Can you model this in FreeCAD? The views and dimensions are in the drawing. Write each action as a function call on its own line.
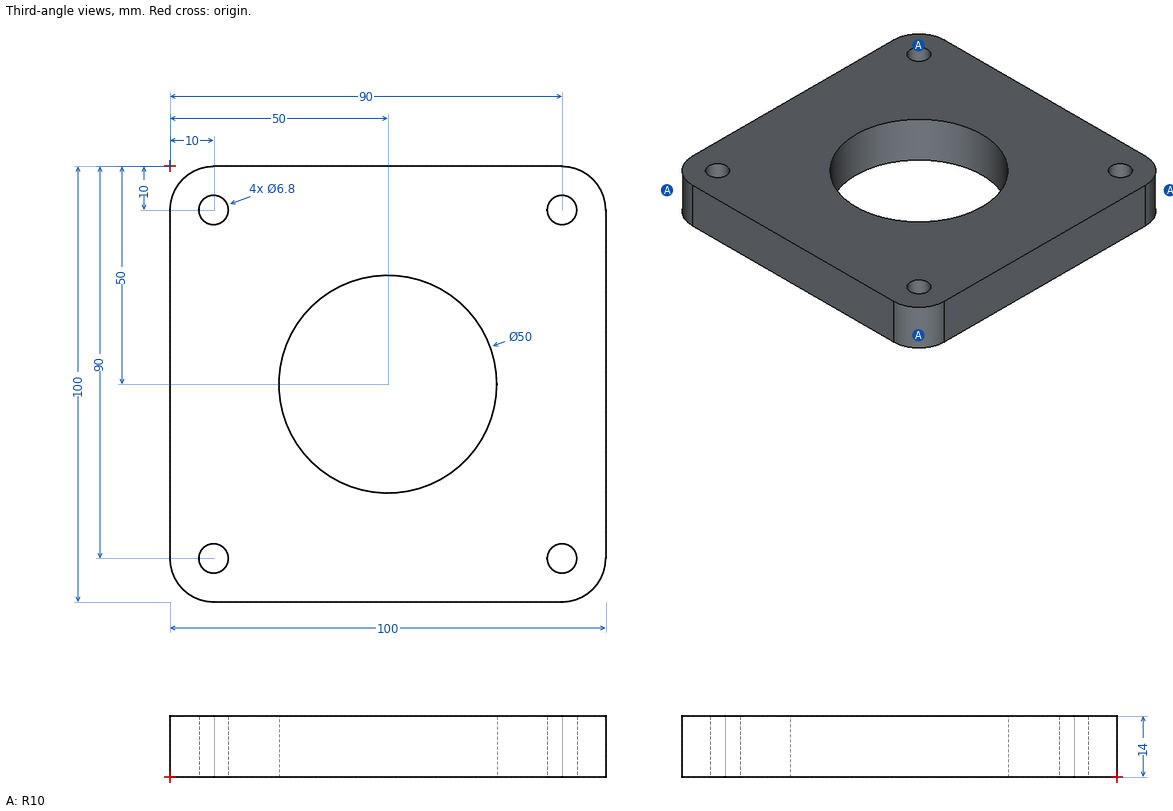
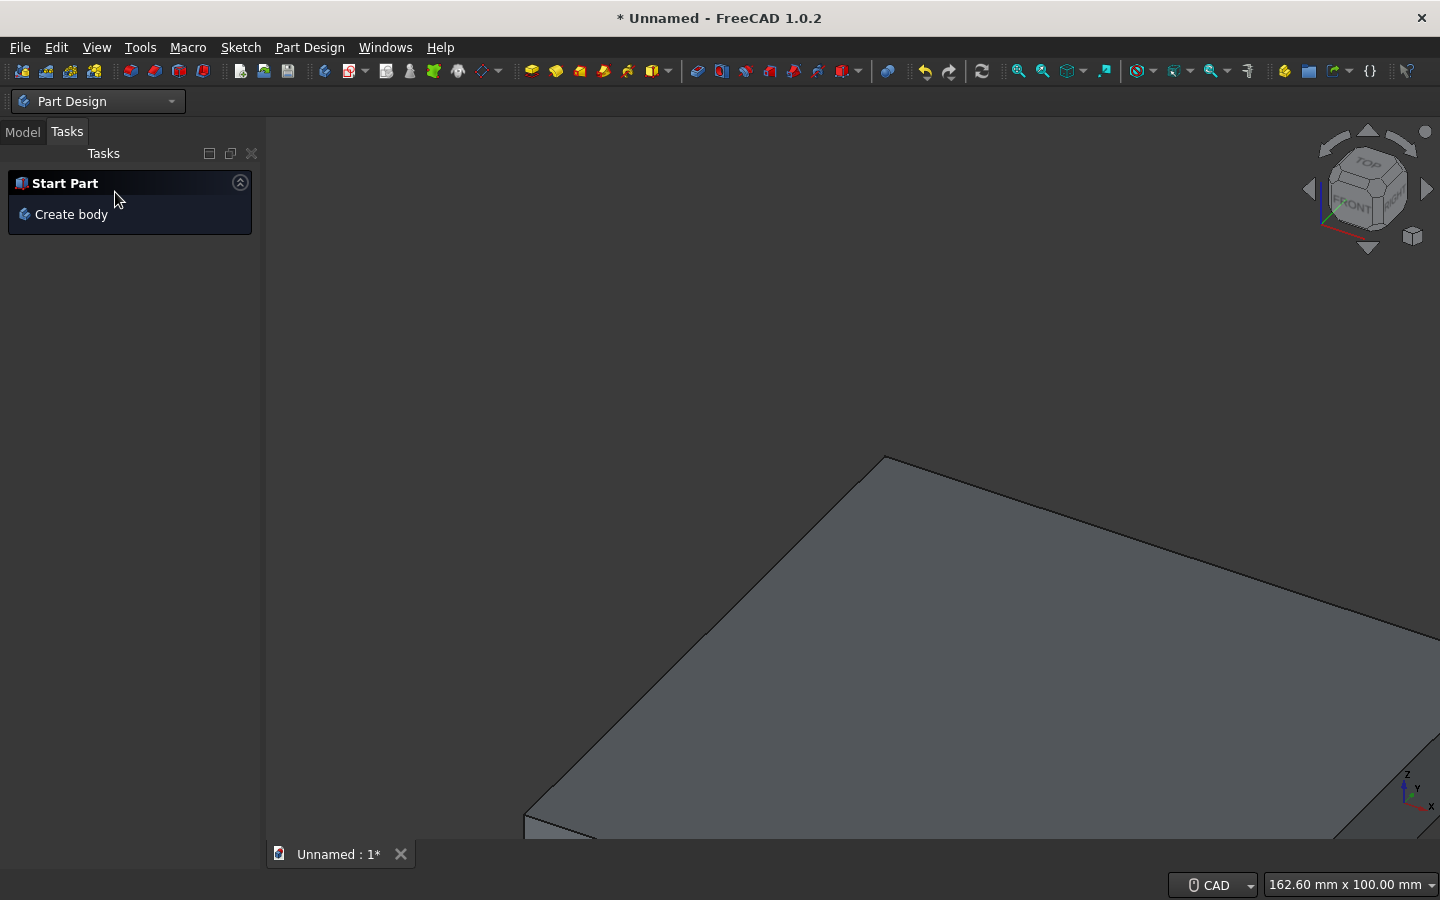
click(1020, 72)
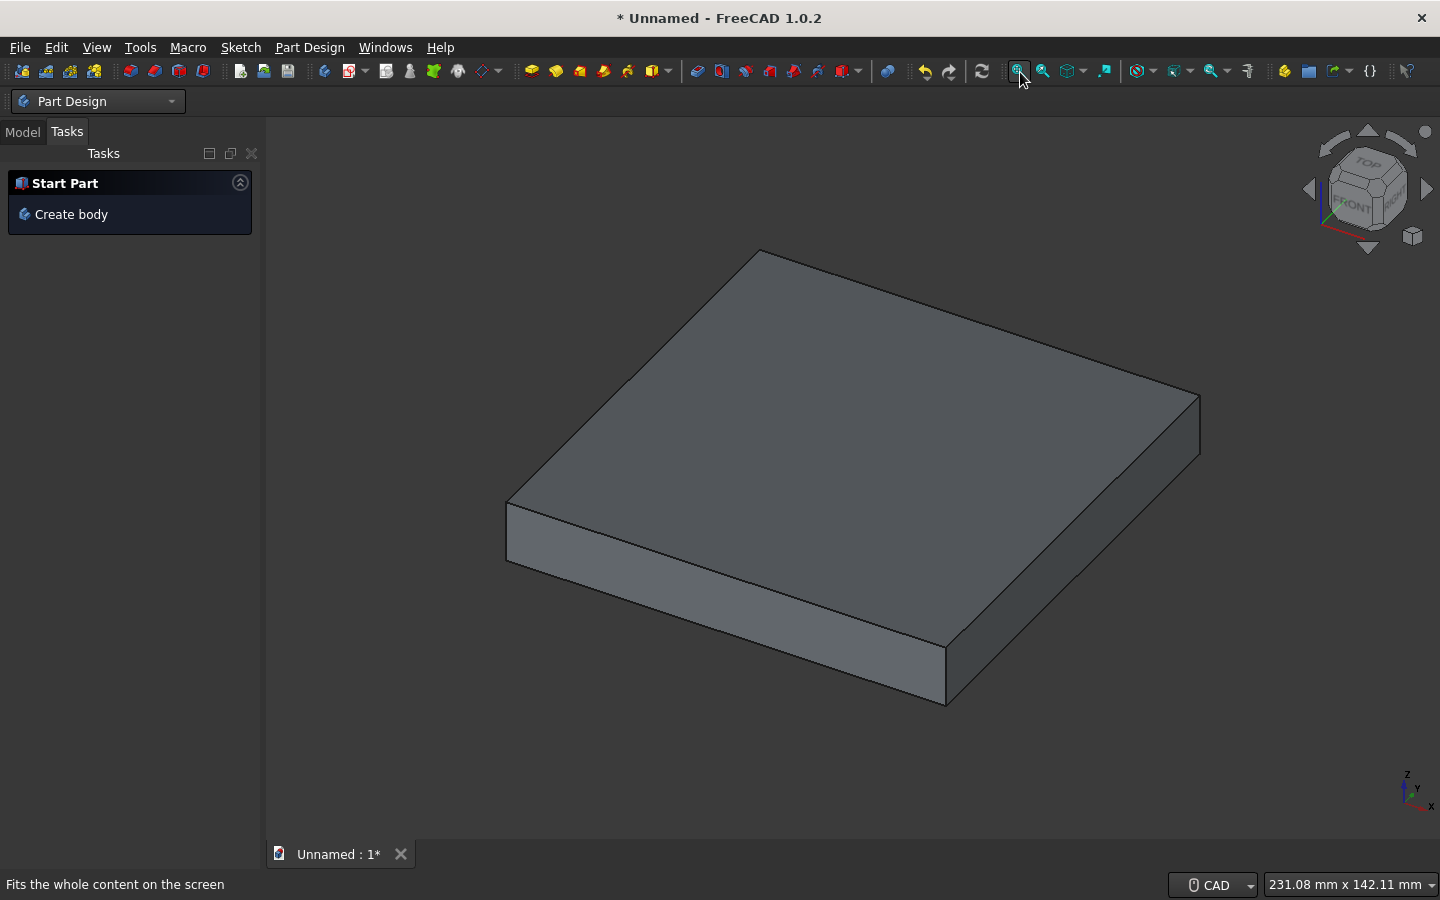
click(853, 448)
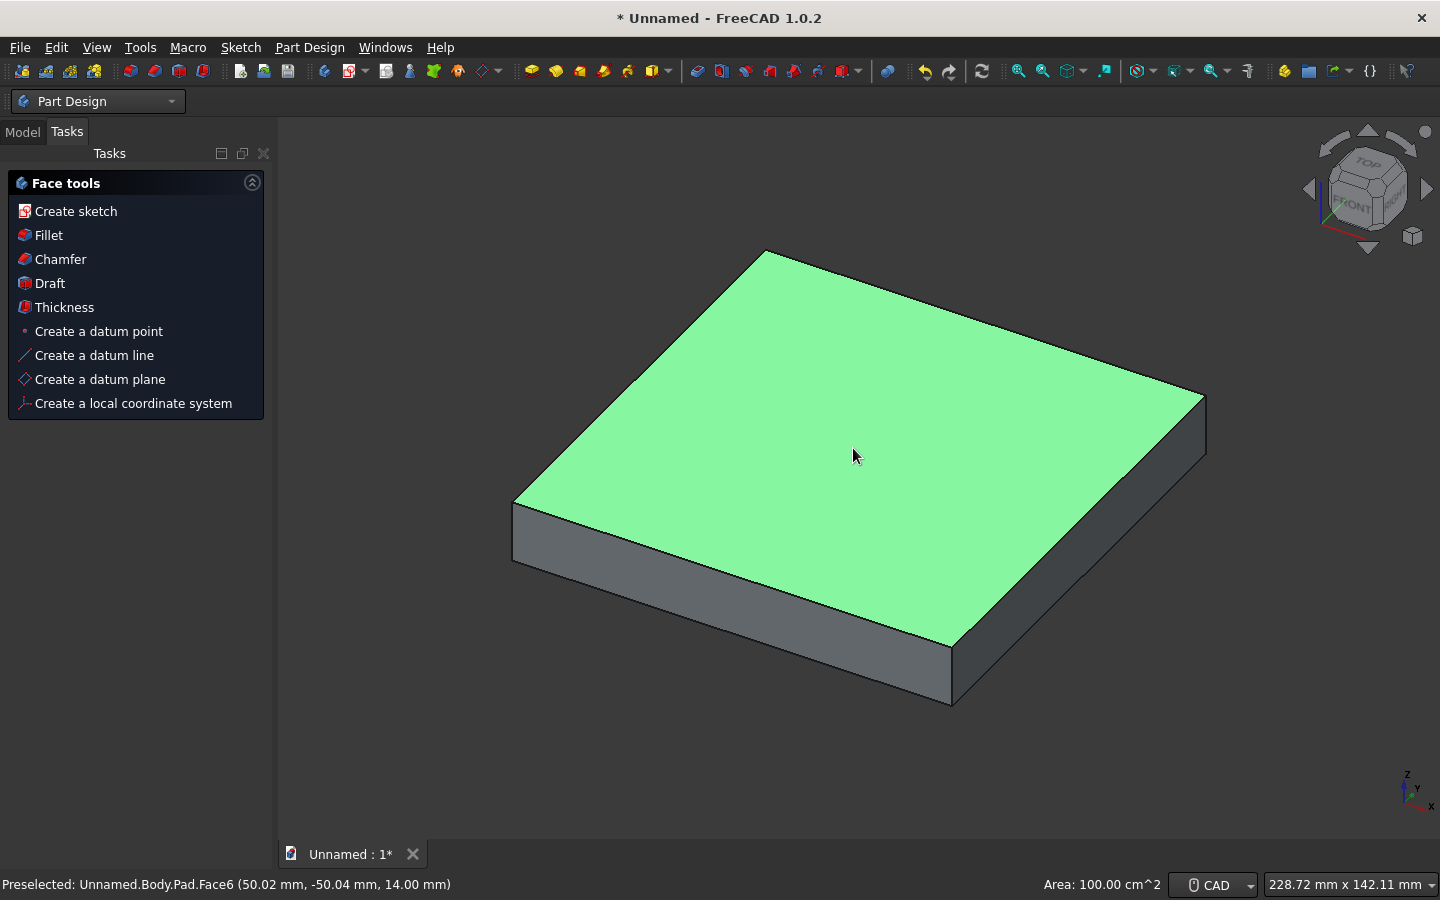
click(350, 72)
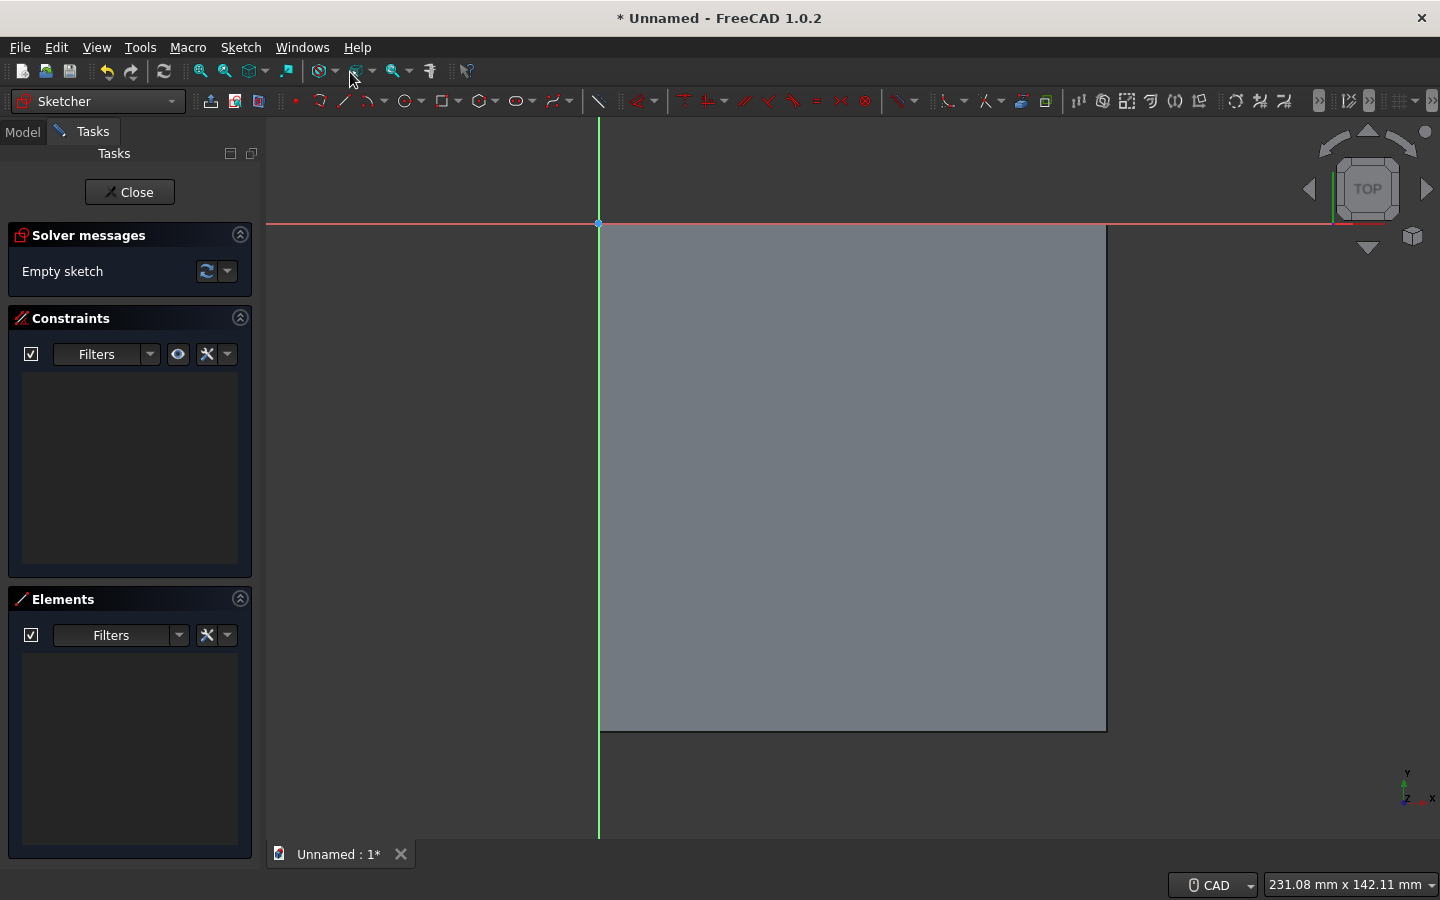
click(406, 102)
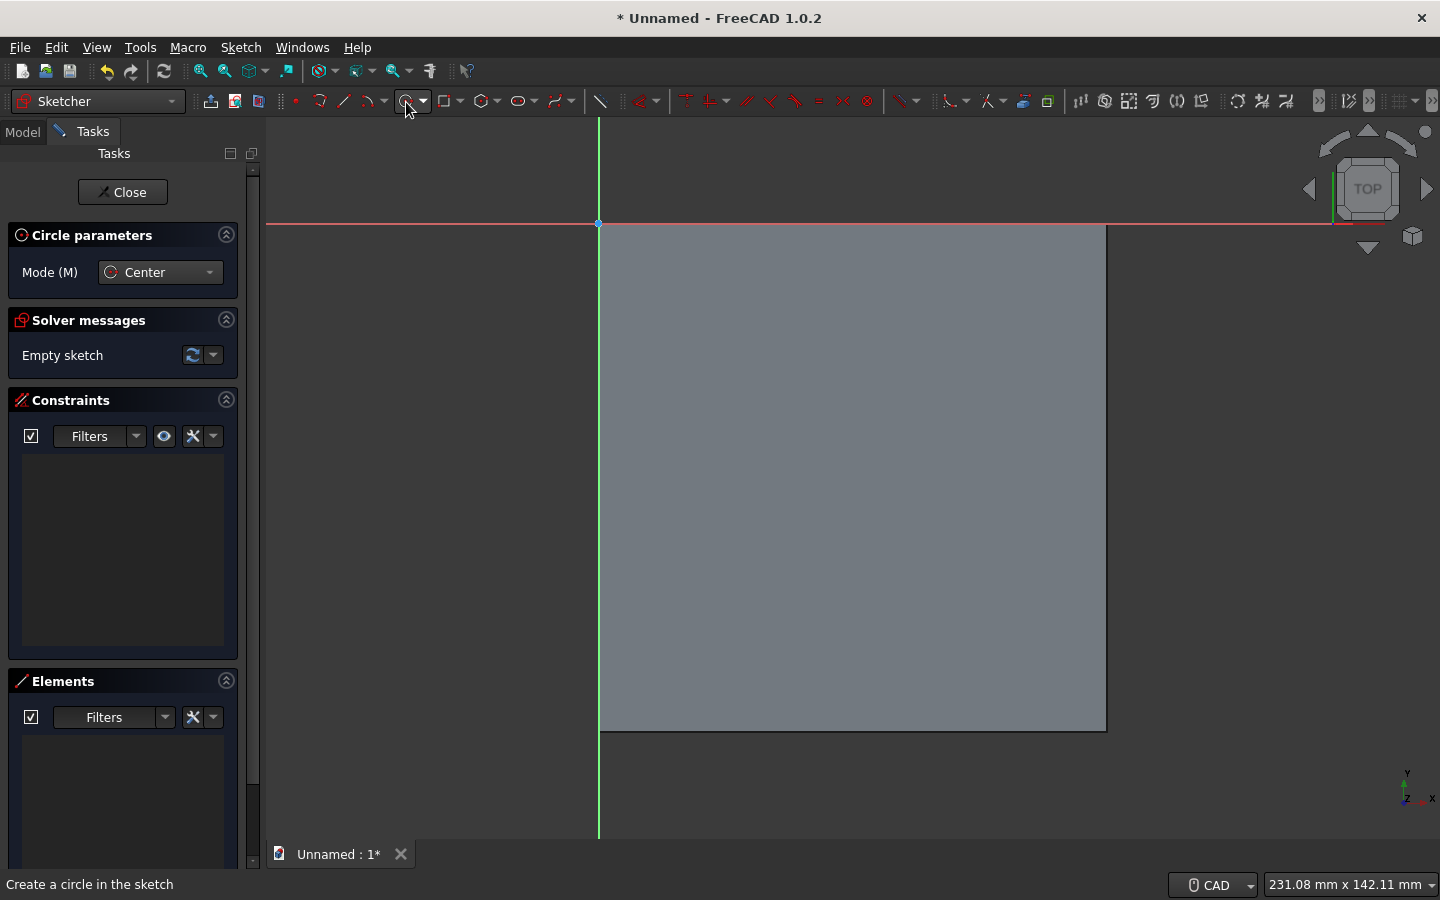
click(853, 478)
click(943, 388)
key(Escape)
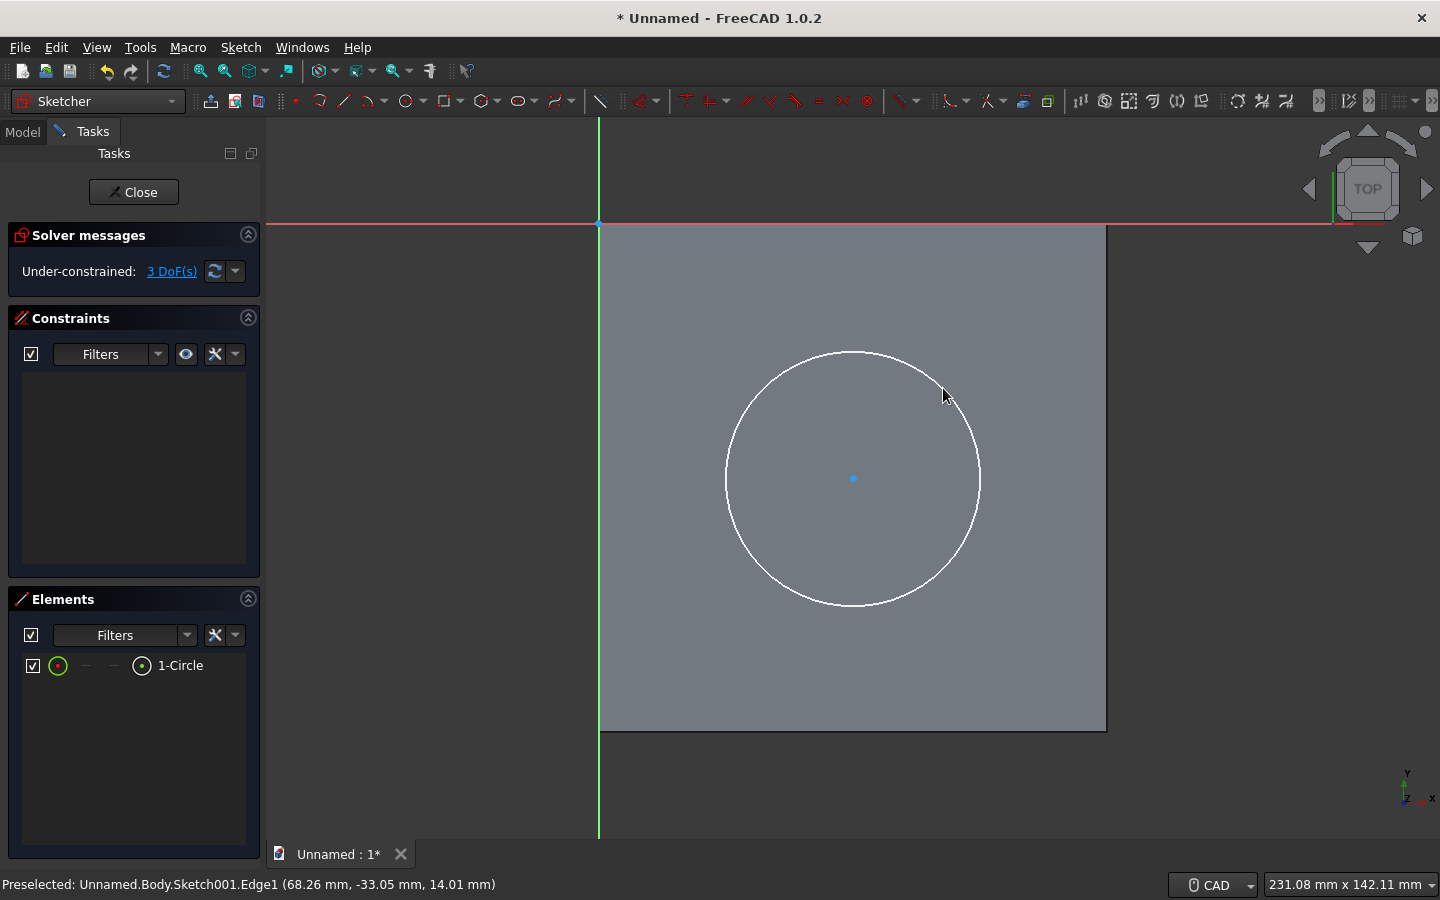
key(d)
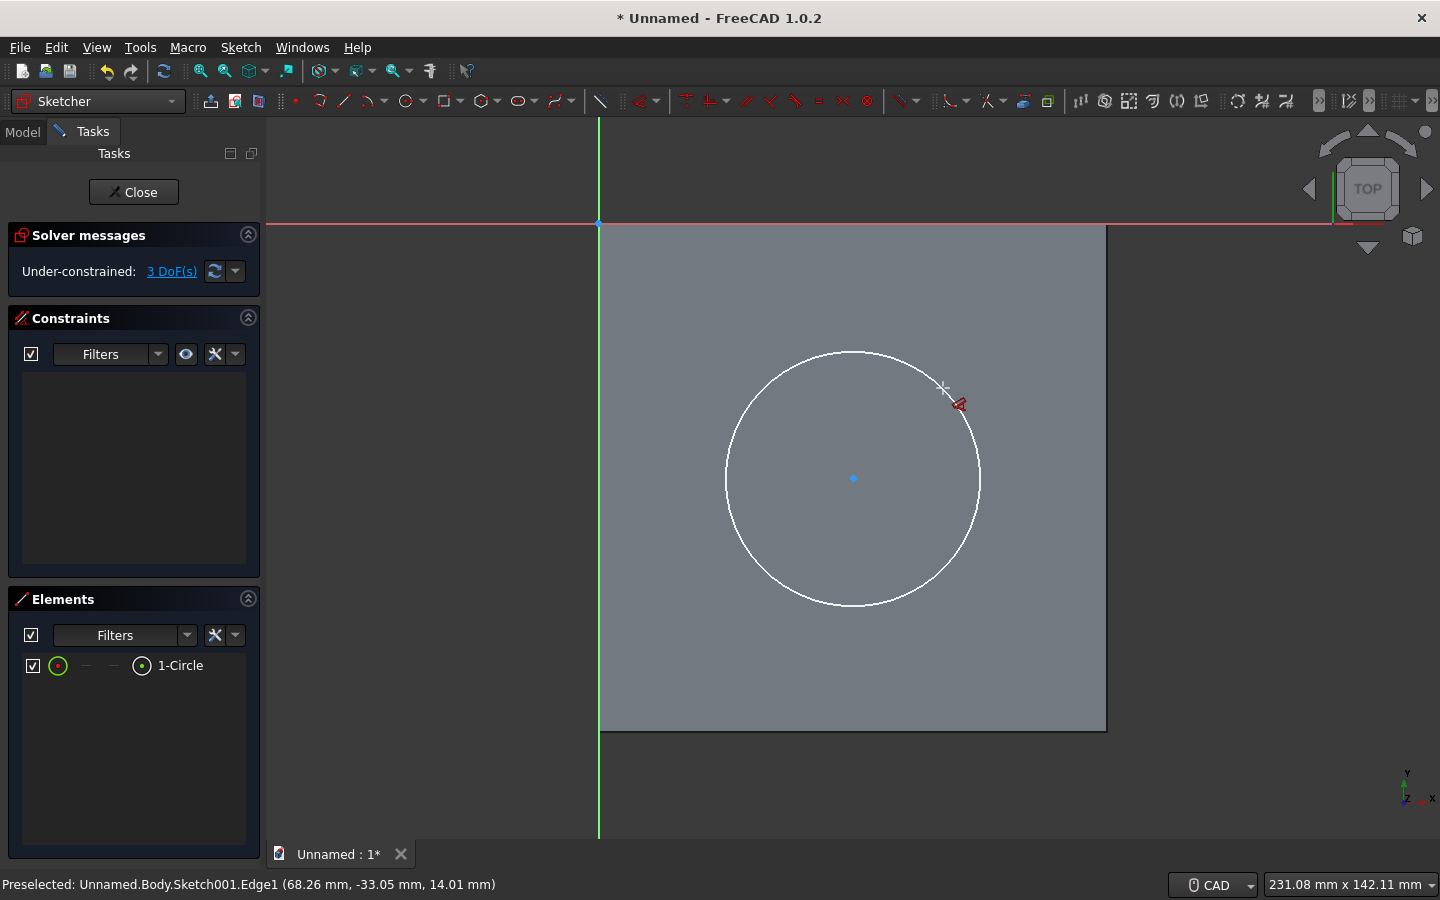
click(943, 389)
click(966, 366)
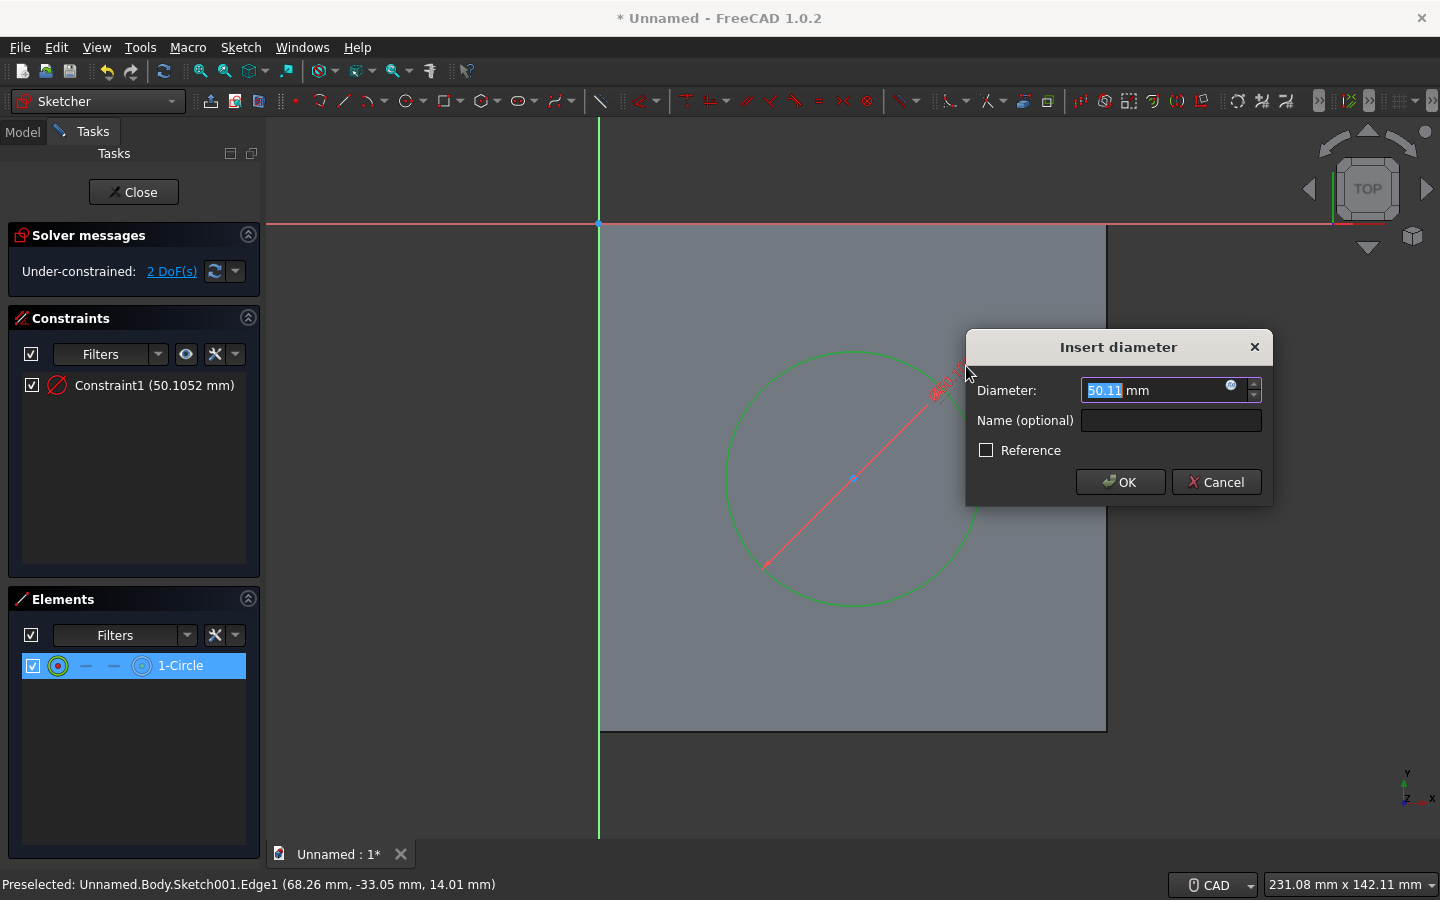
text(50)
key(Return)